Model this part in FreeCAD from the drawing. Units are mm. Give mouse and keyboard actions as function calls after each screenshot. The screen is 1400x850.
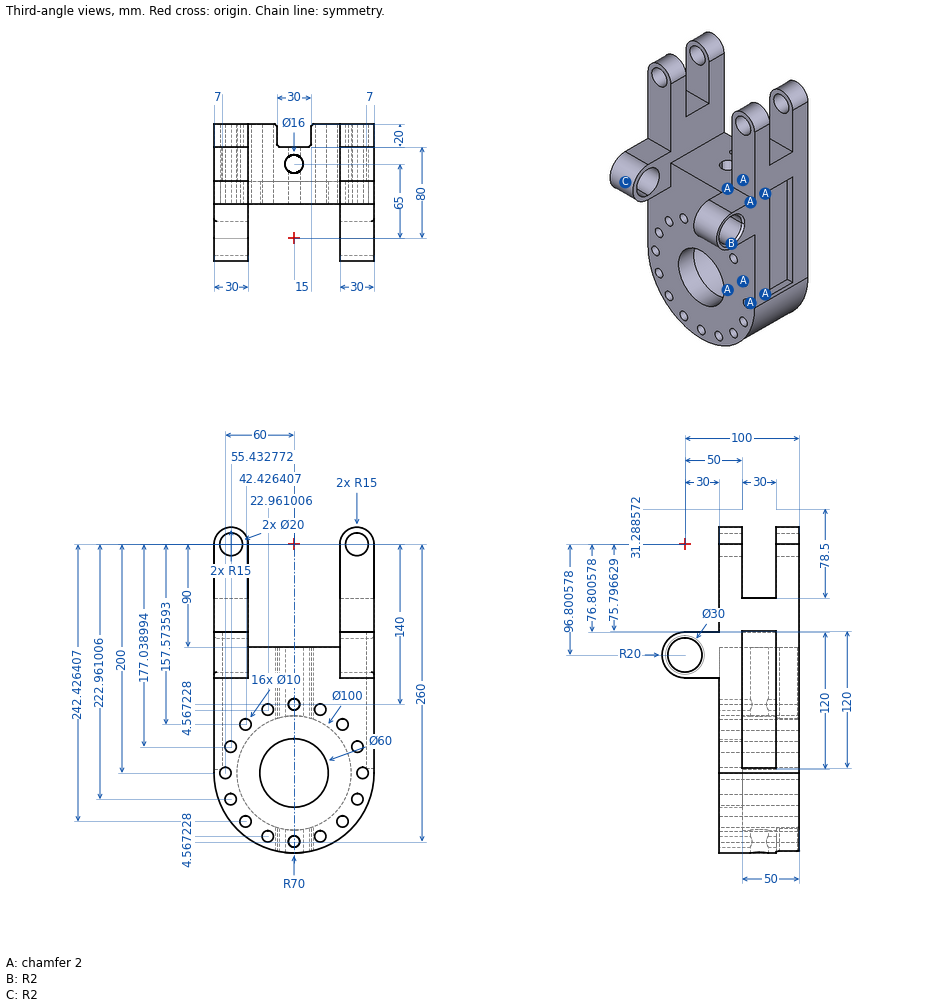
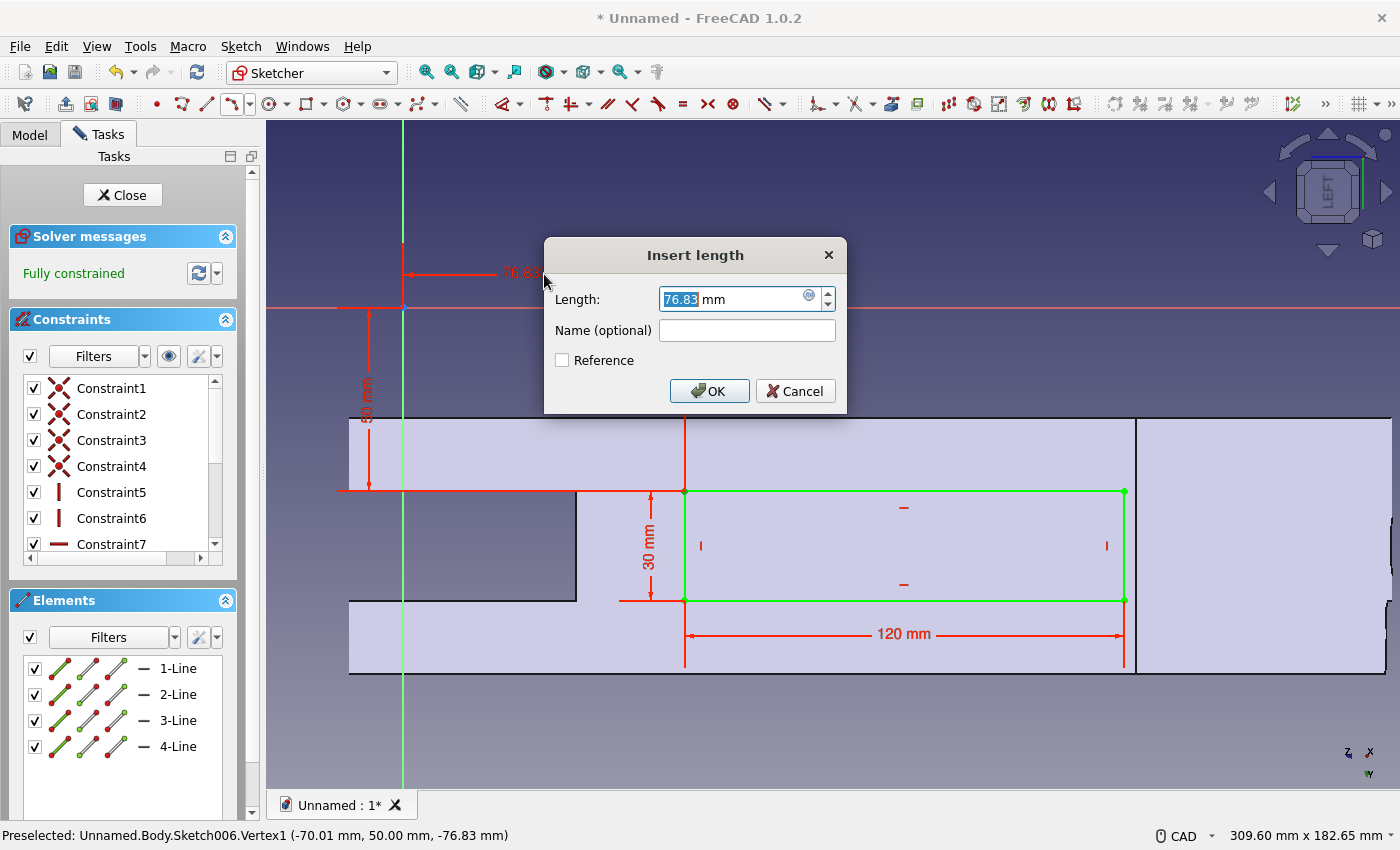
text(76.800578)
key(Return)
key(Escape)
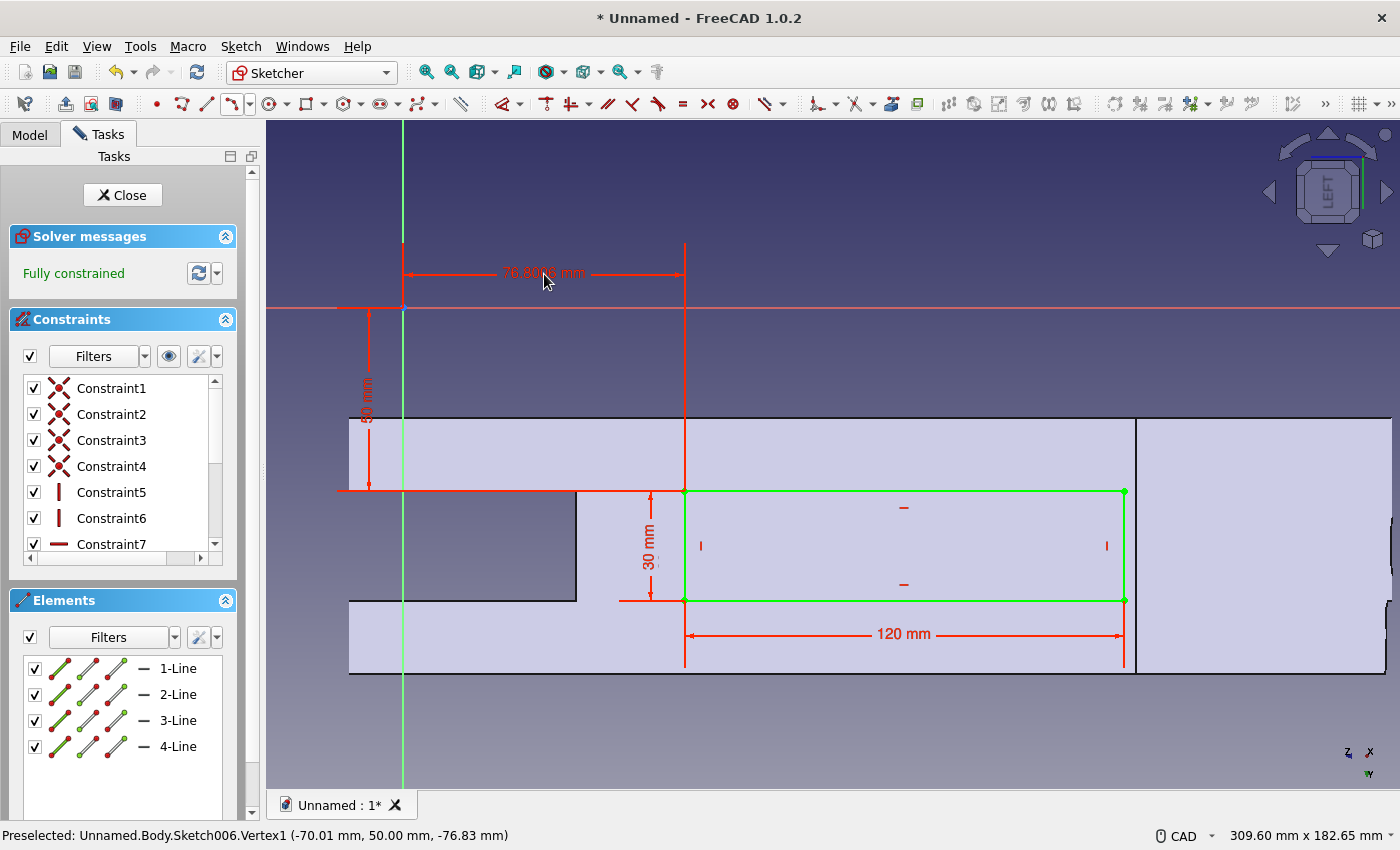
click(123, 195)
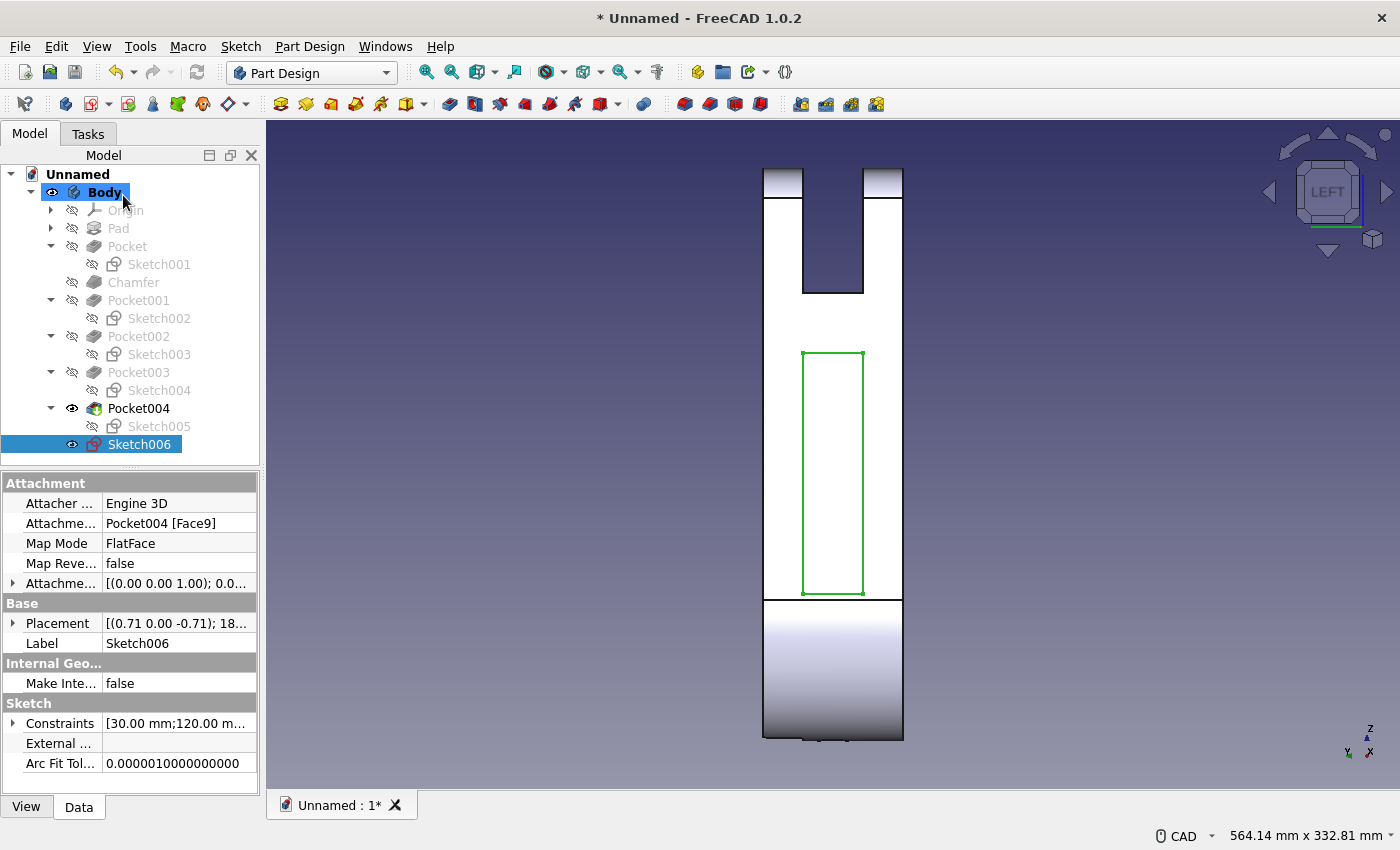
click(450, 104)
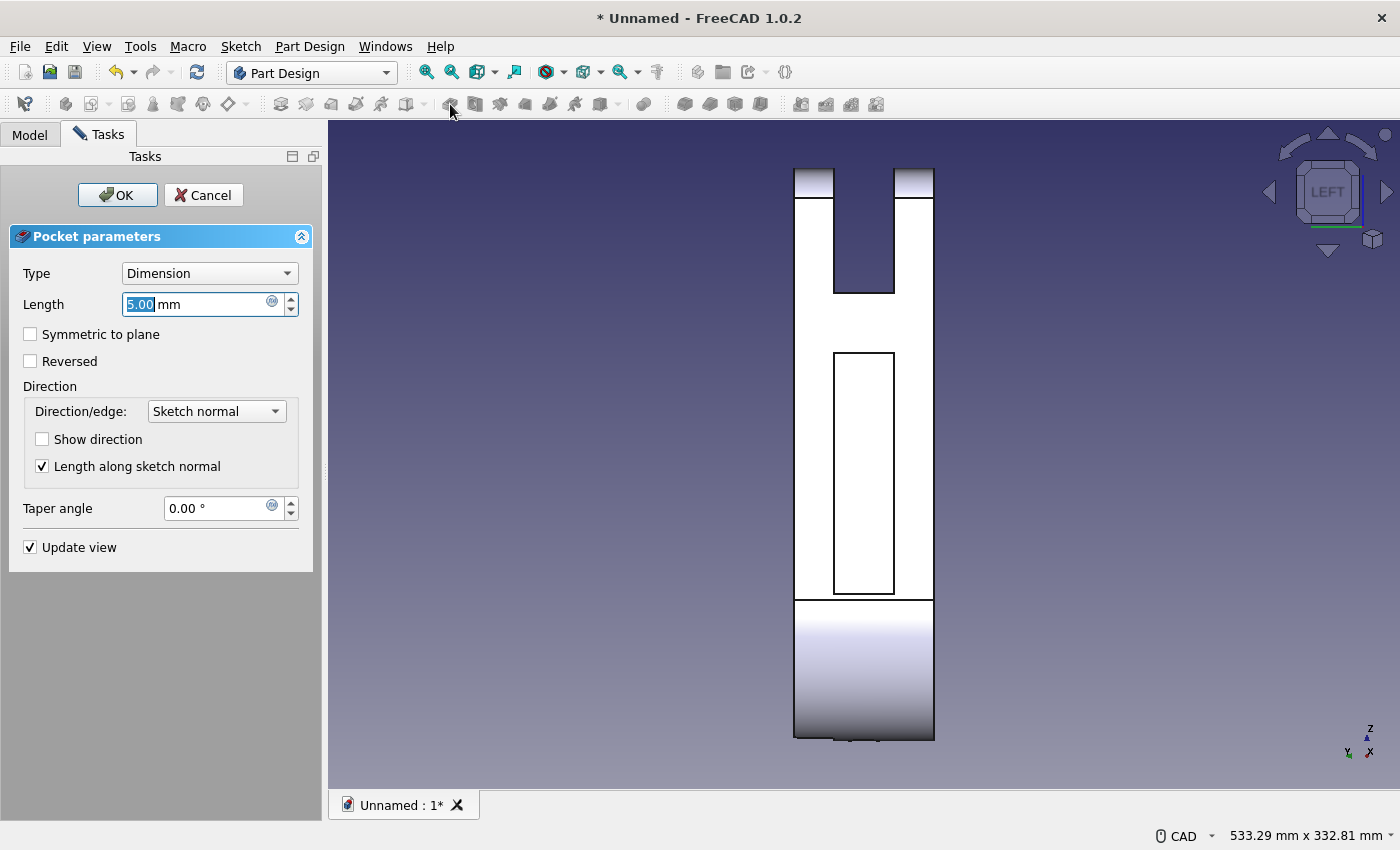
text(7)
key(Tab)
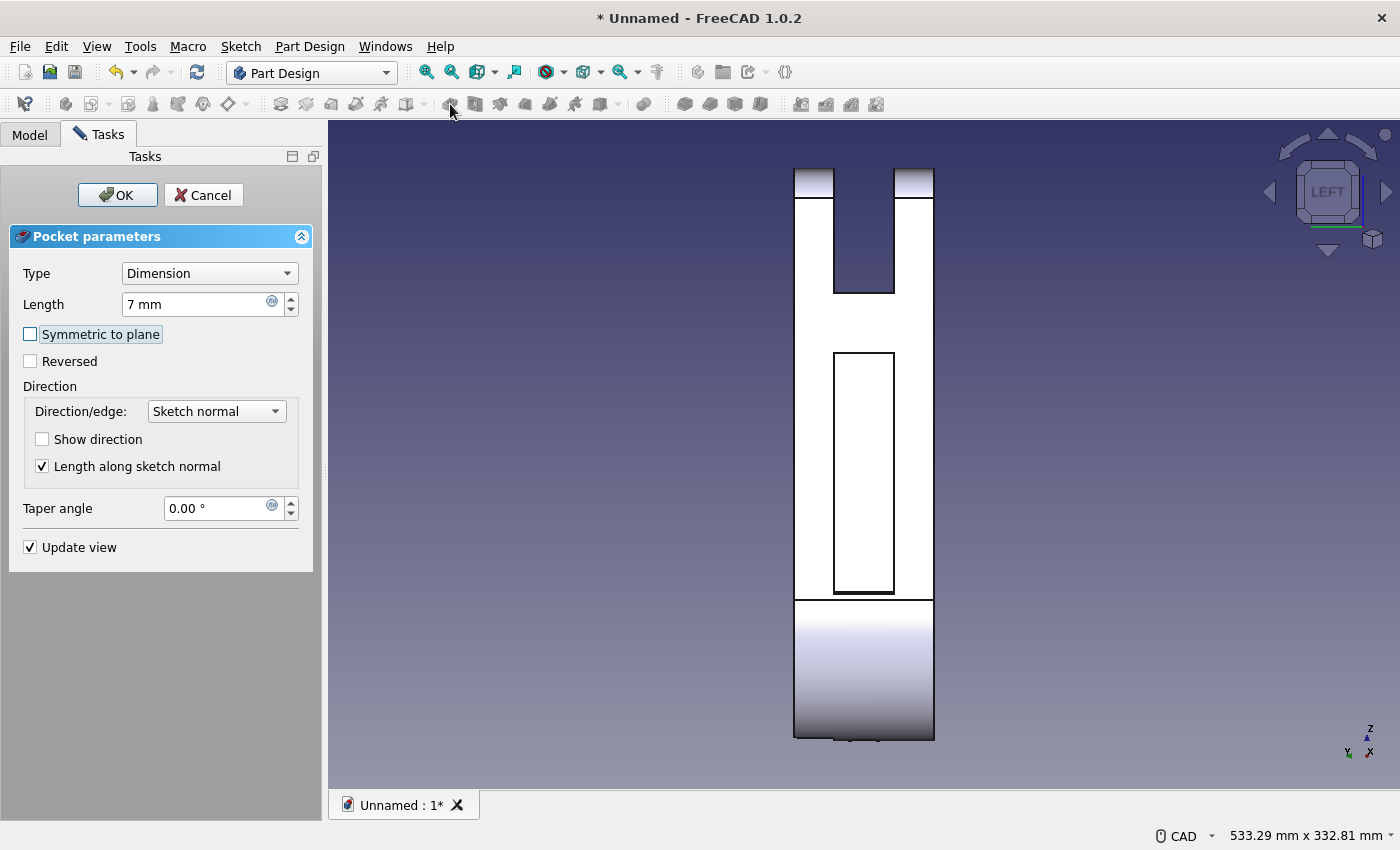
click(118, 195)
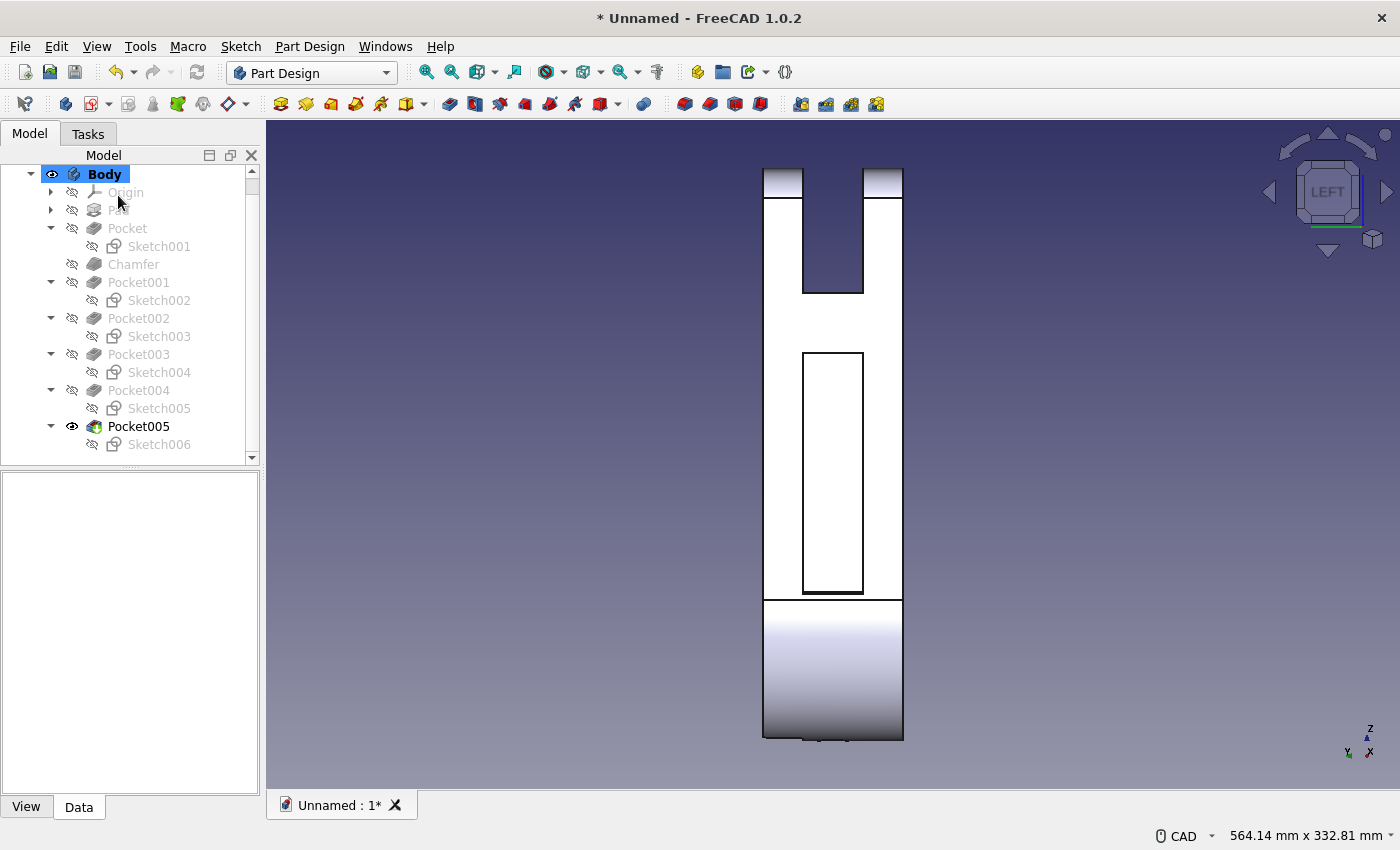
key(0)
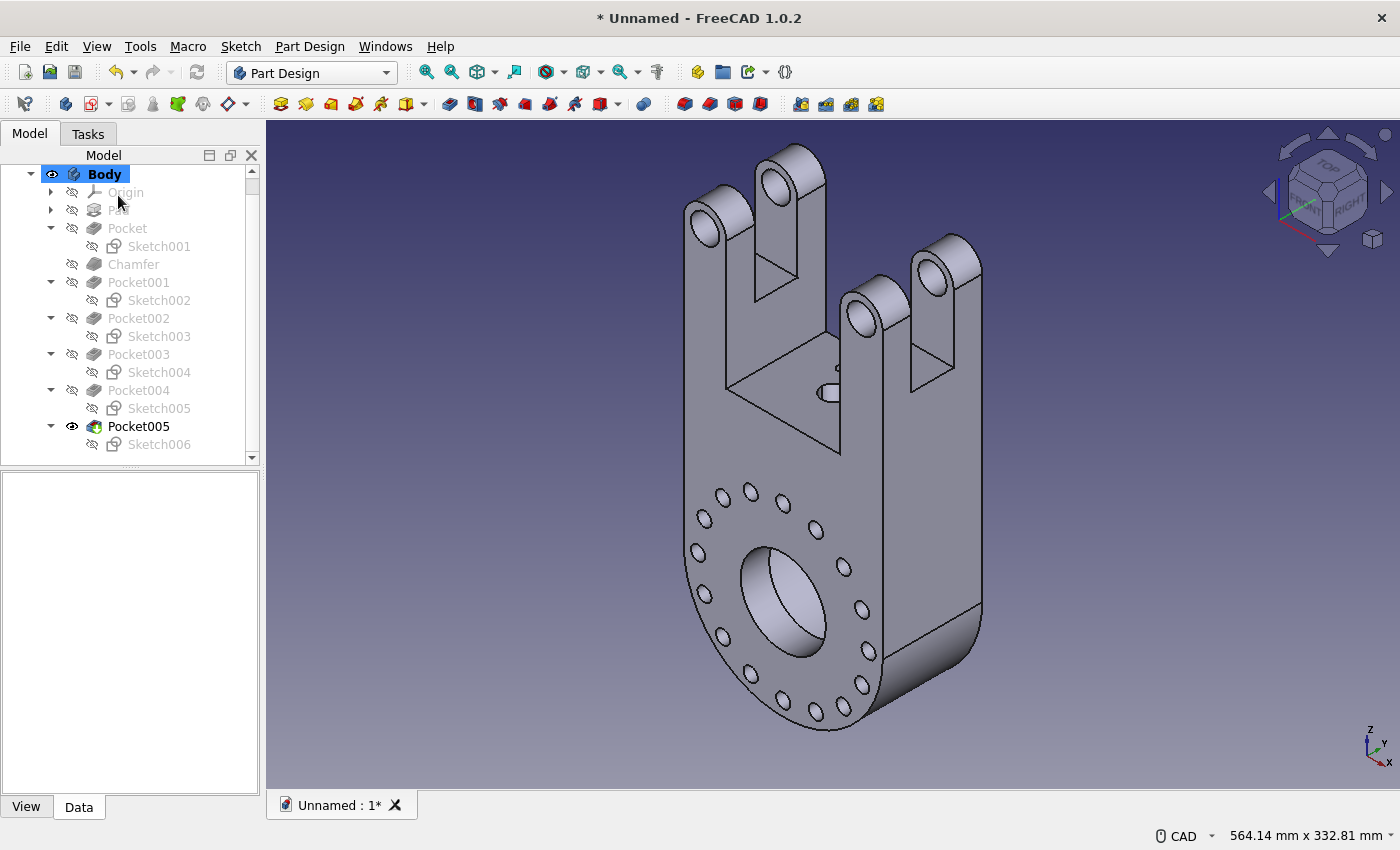
click(933, 513)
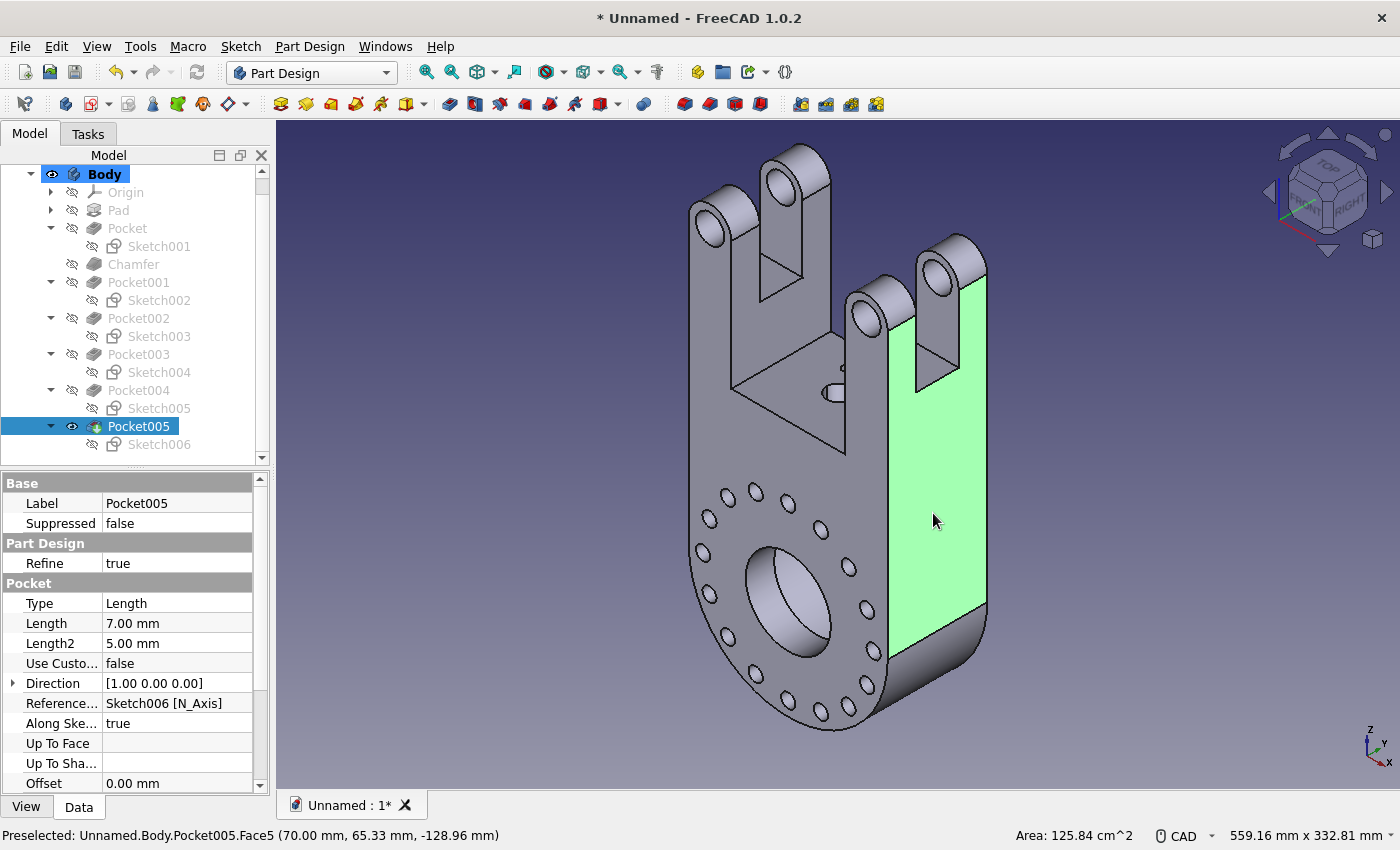
click(90, 104)